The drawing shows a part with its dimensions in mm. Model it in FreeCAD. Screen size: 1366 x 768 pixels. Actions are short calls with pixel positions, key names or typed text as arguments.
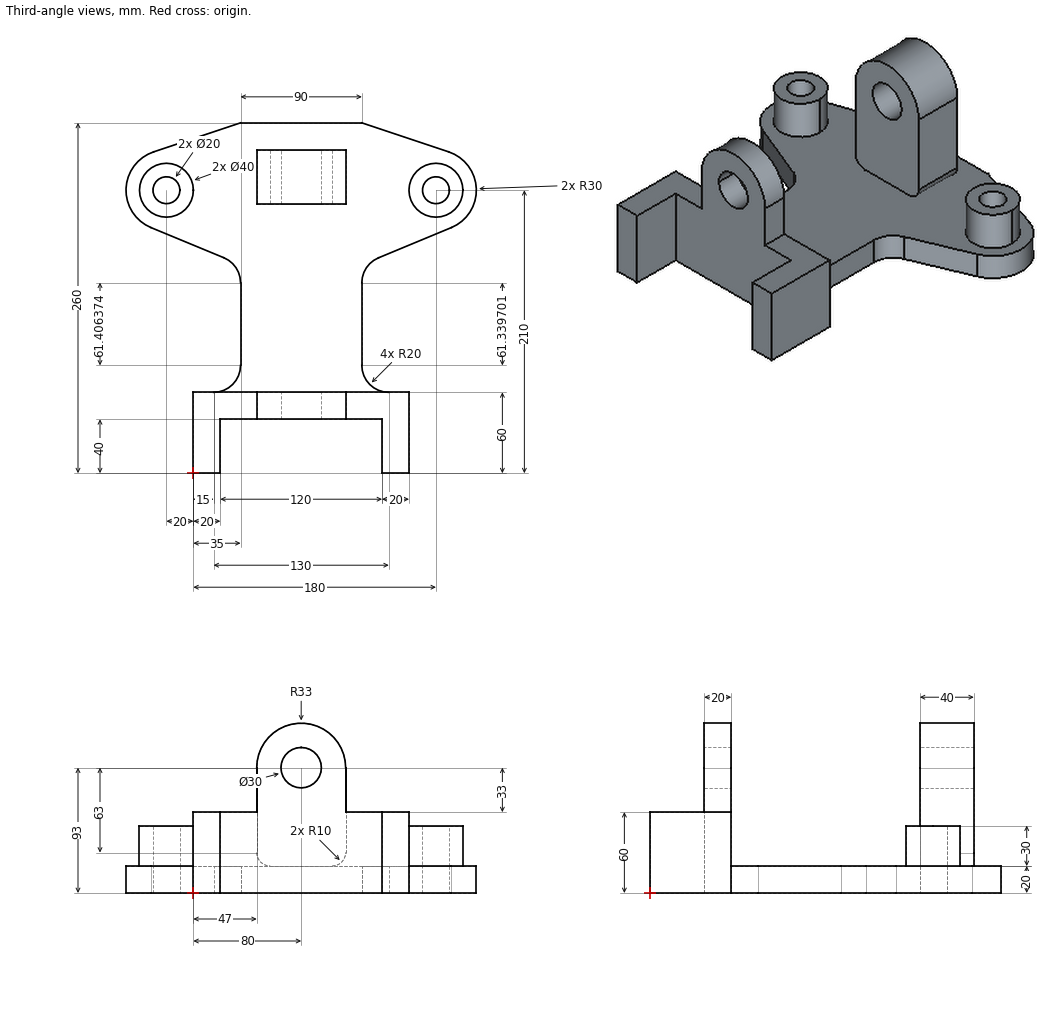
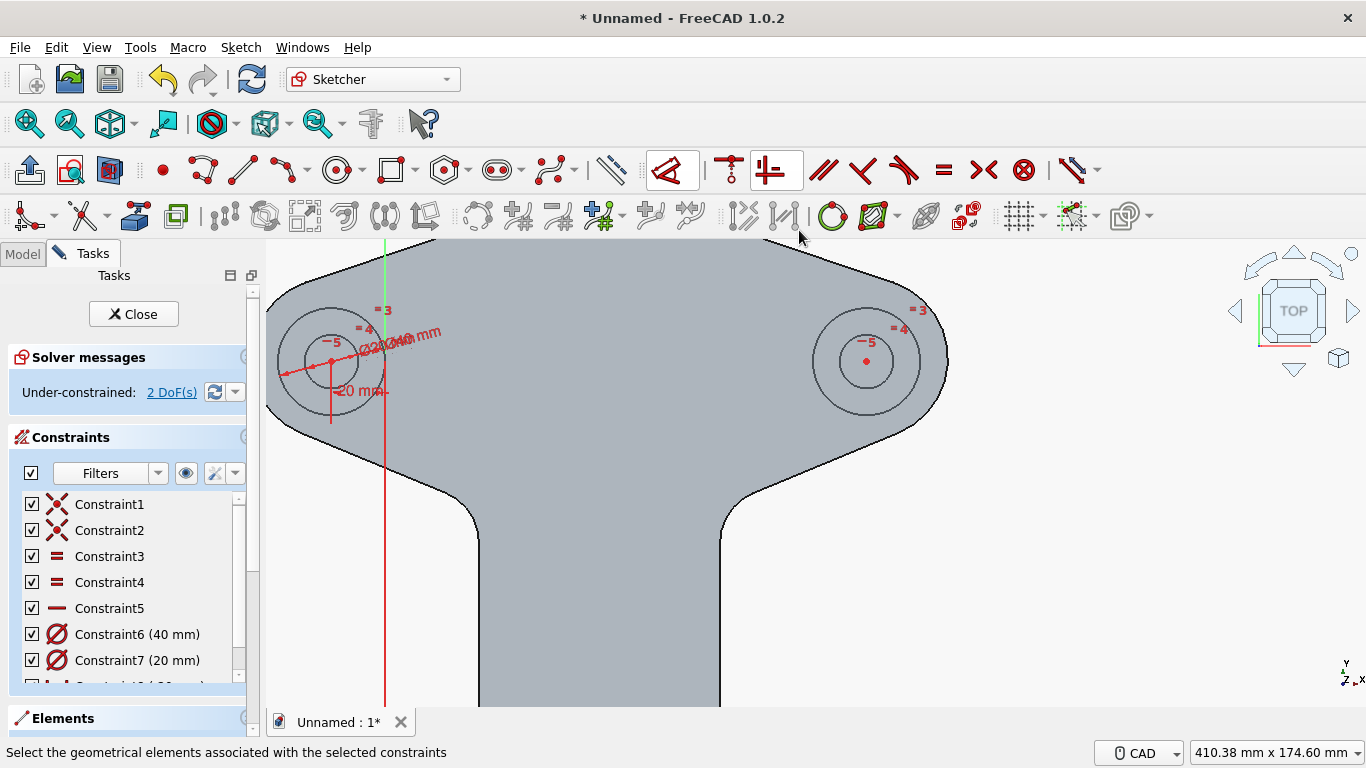
click(331, 362)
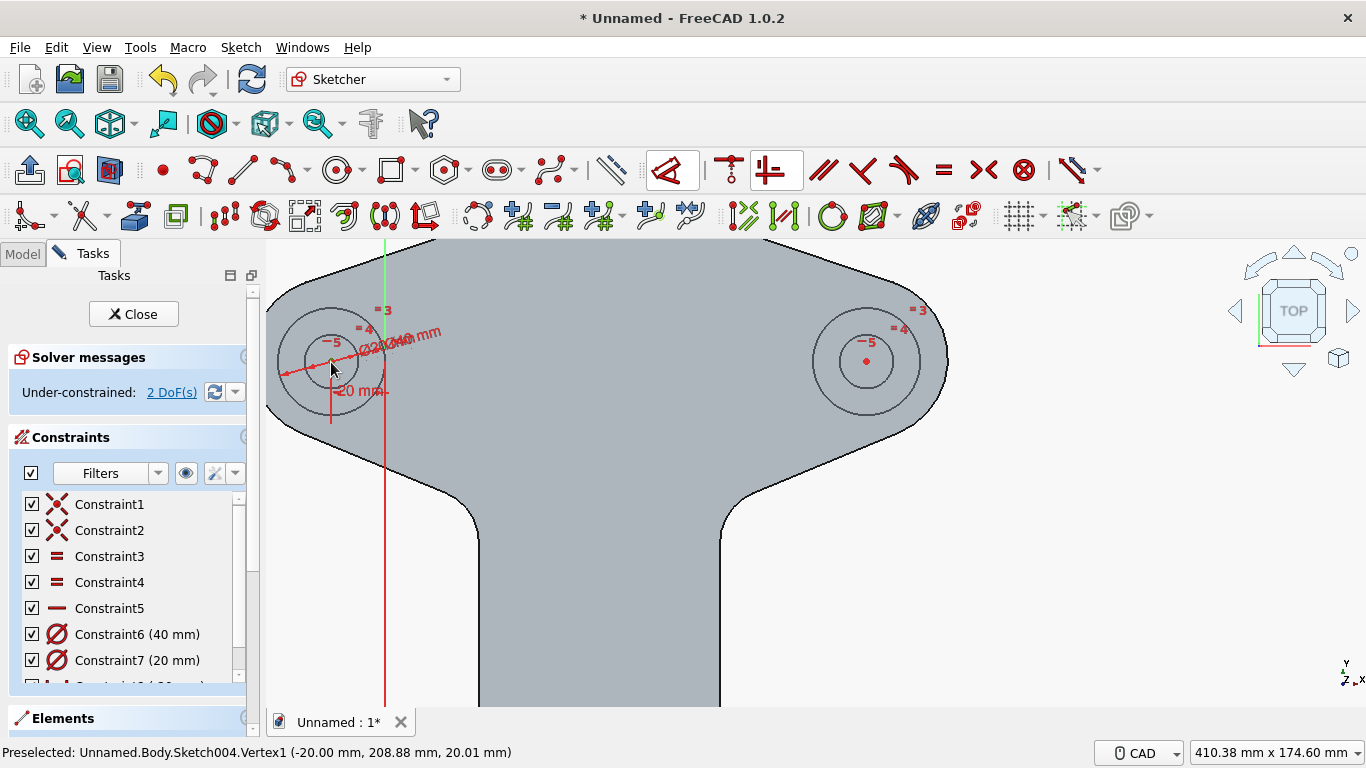
key(i)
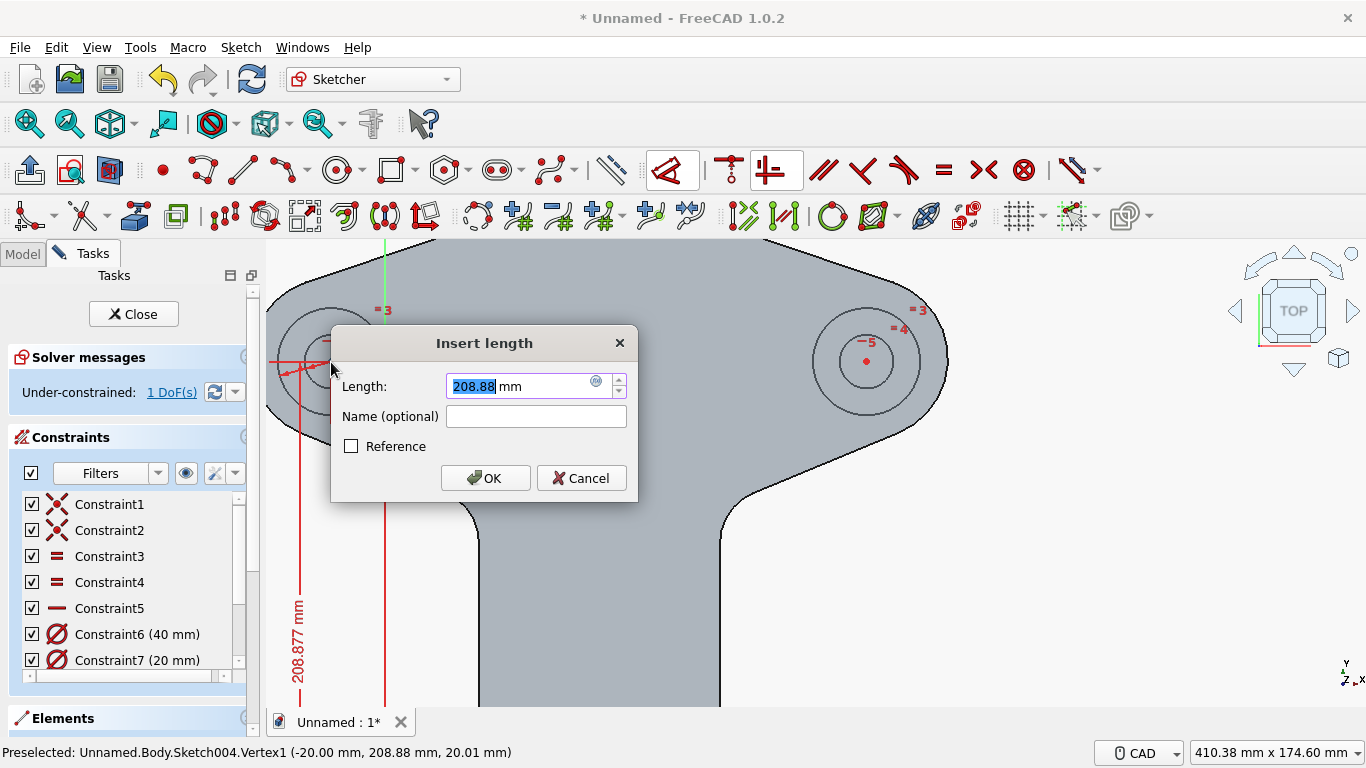
text(210)
key(Return)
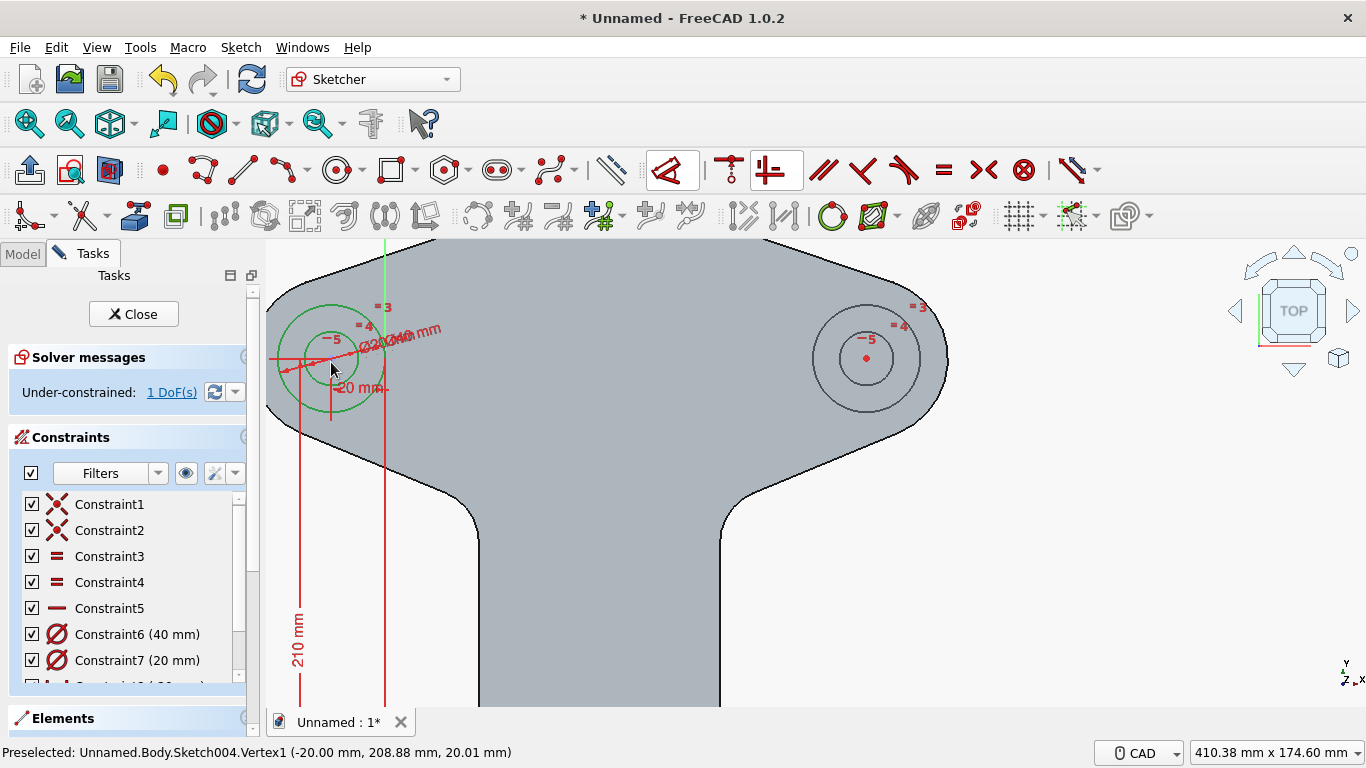
click(867, 359)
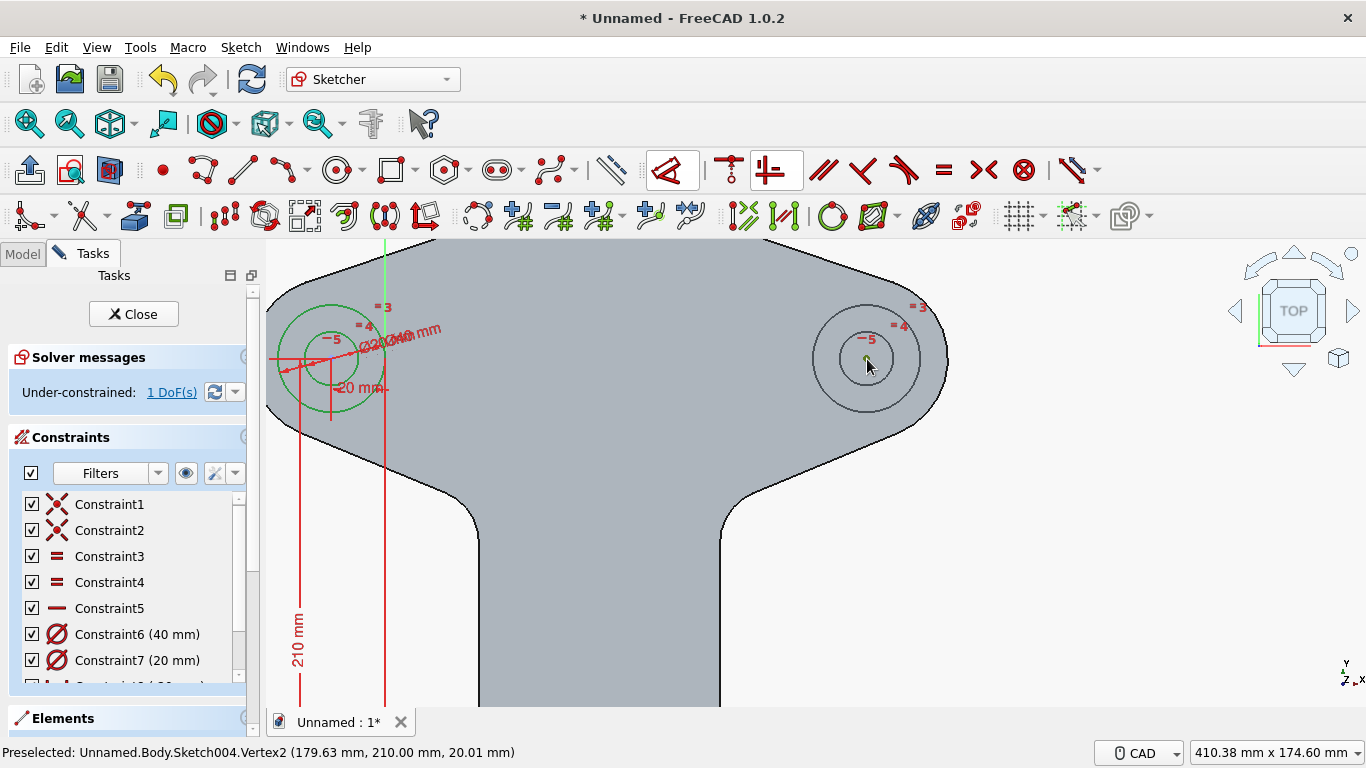
click(694, 170)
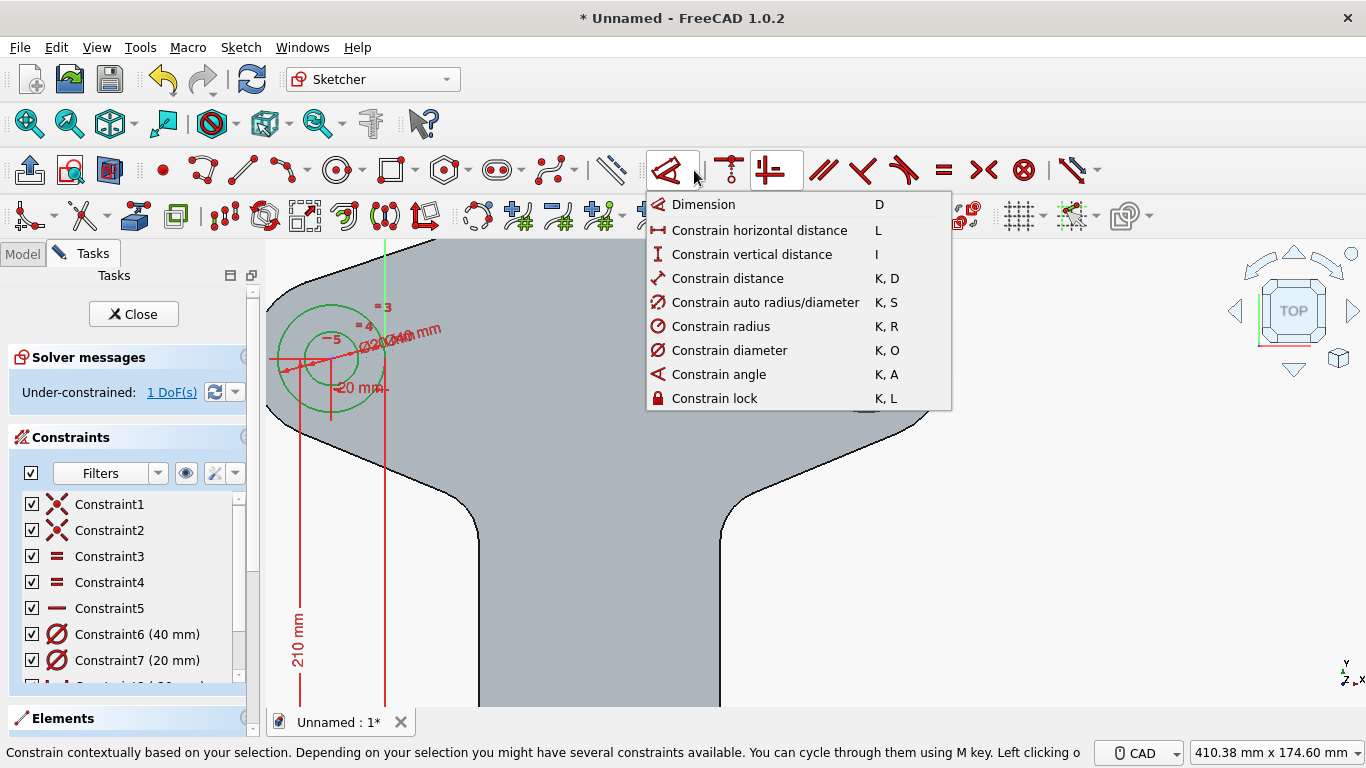
click(799, 230)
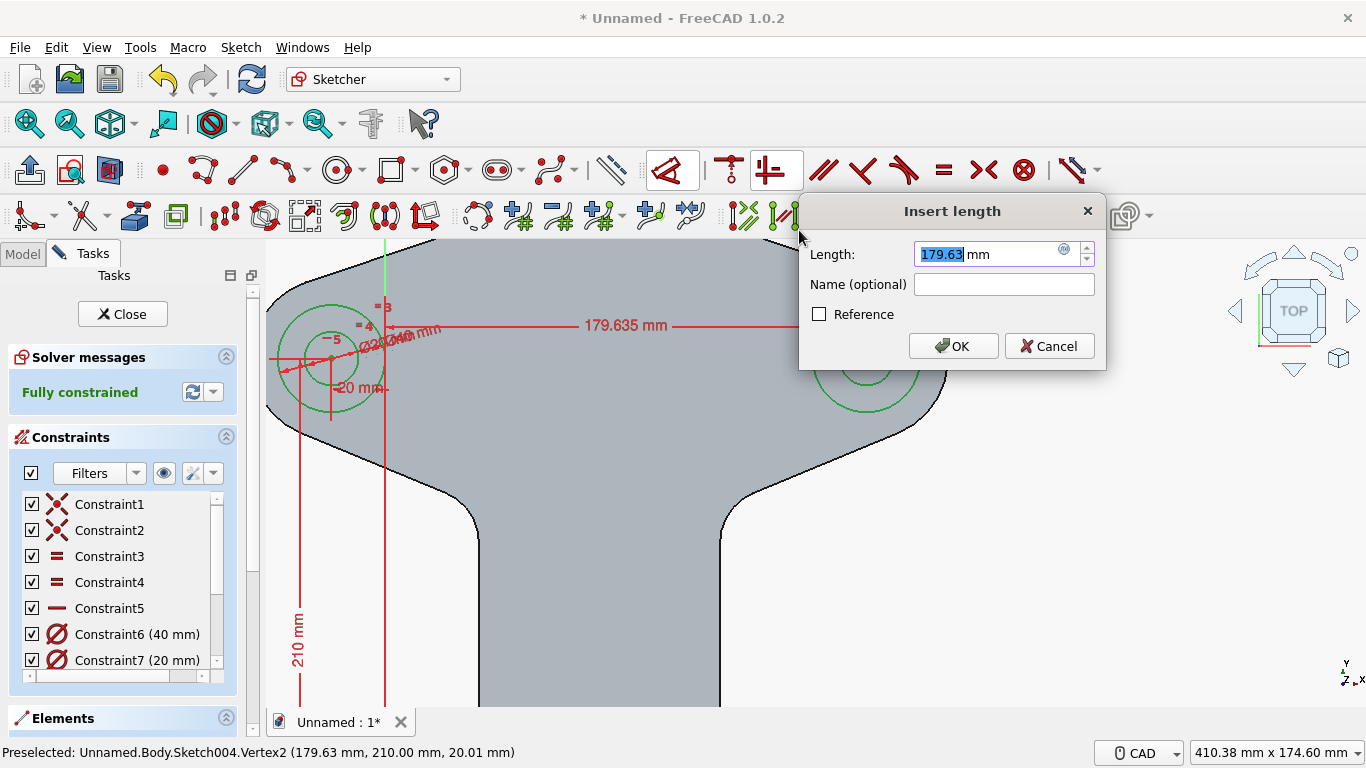
text(180)
key(Return)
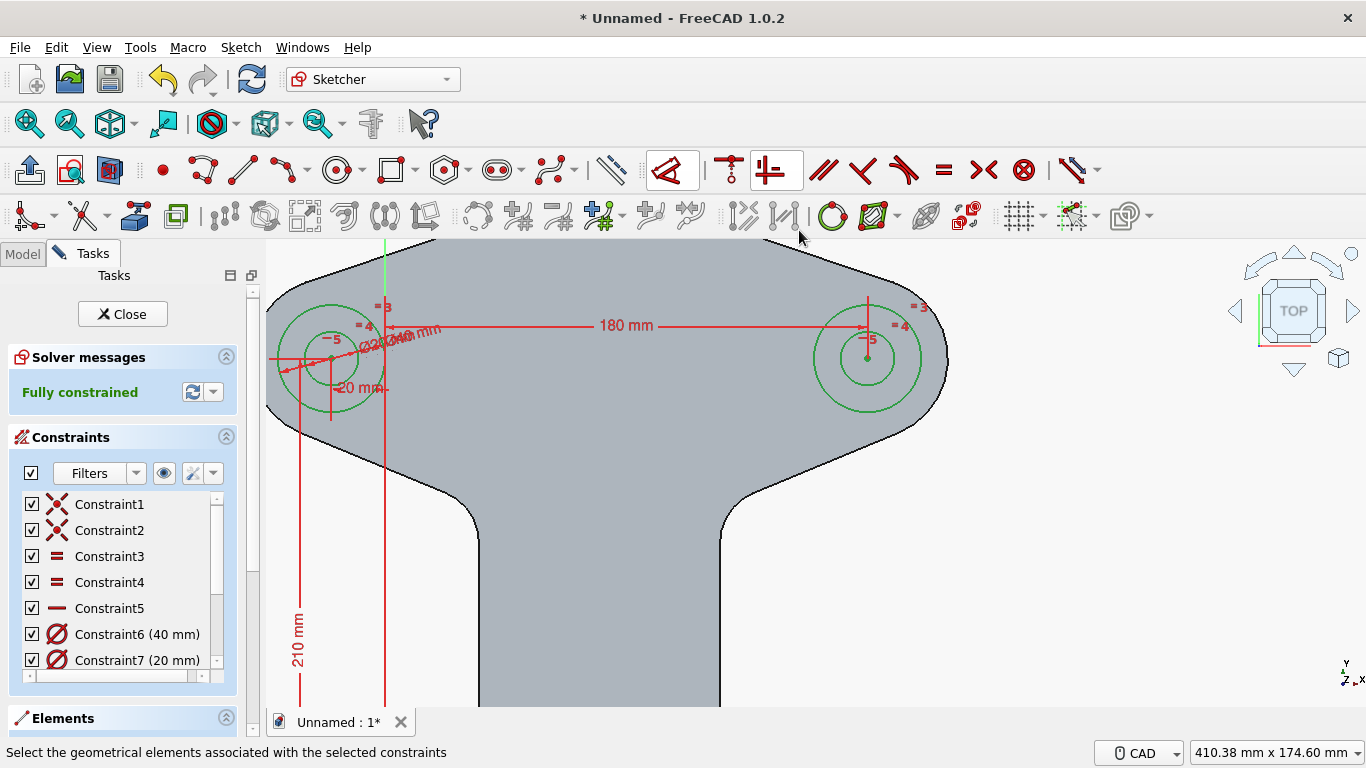
click(123, 314)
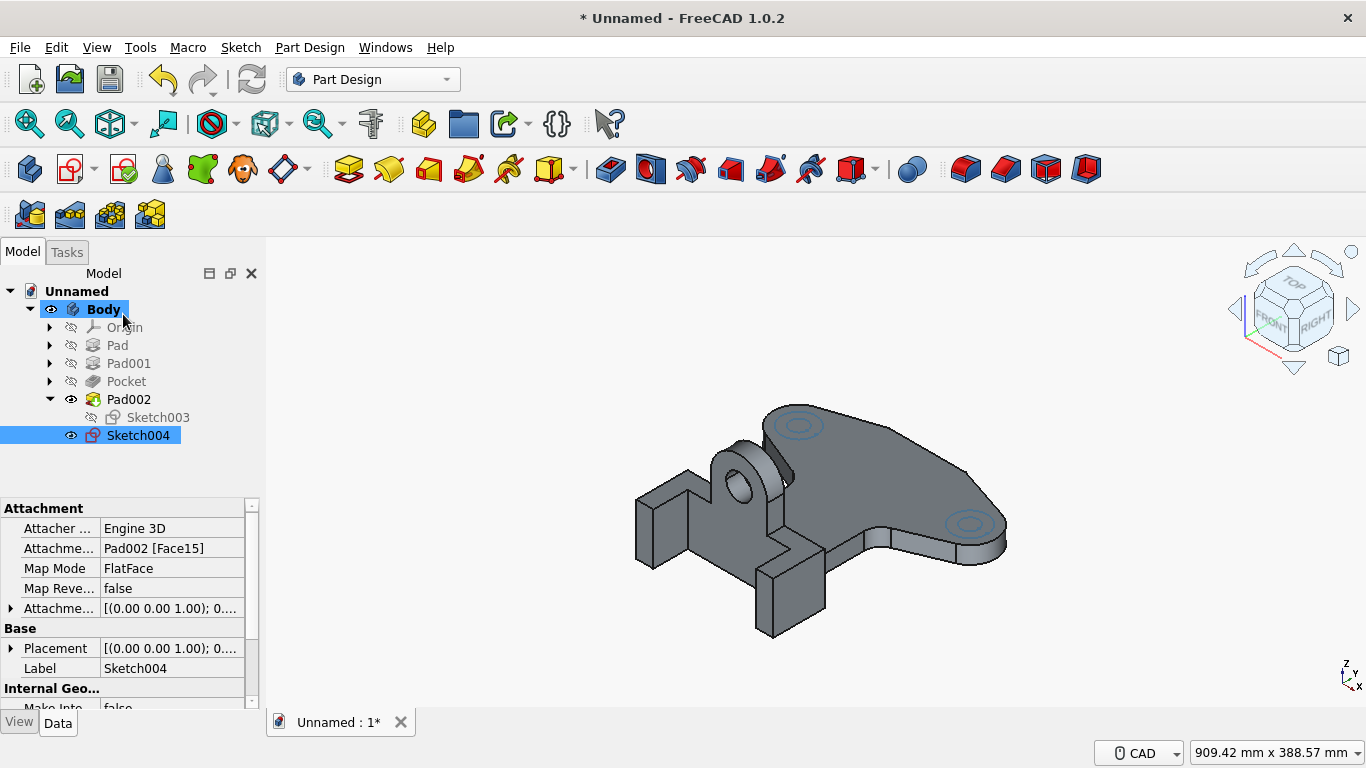
click(350, 170)